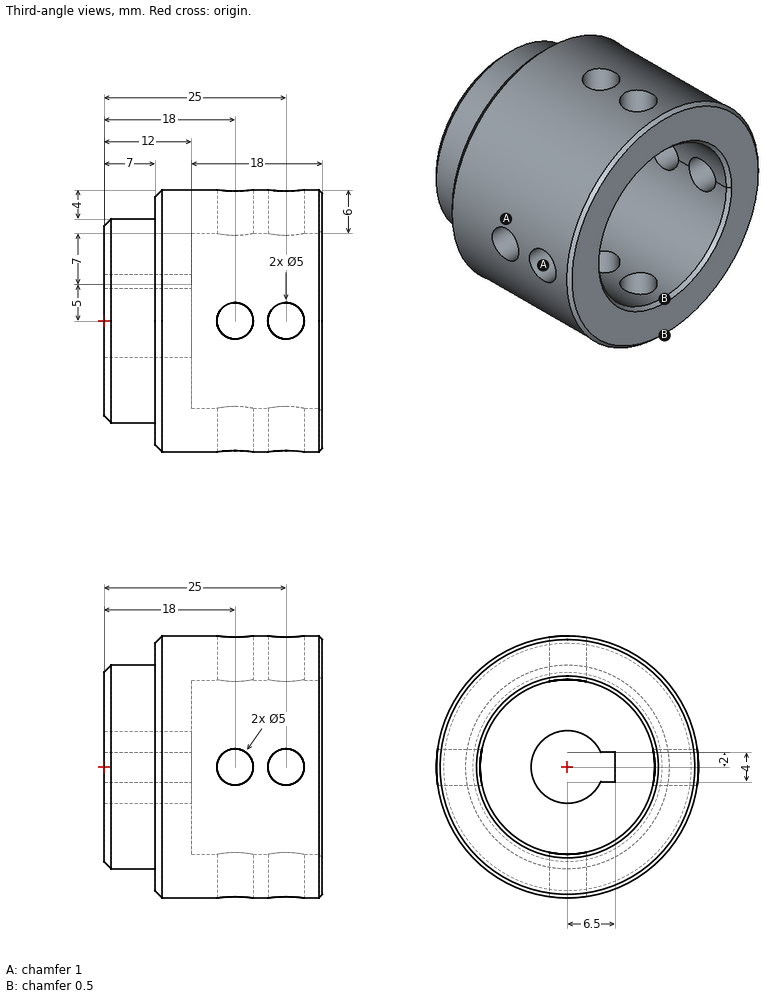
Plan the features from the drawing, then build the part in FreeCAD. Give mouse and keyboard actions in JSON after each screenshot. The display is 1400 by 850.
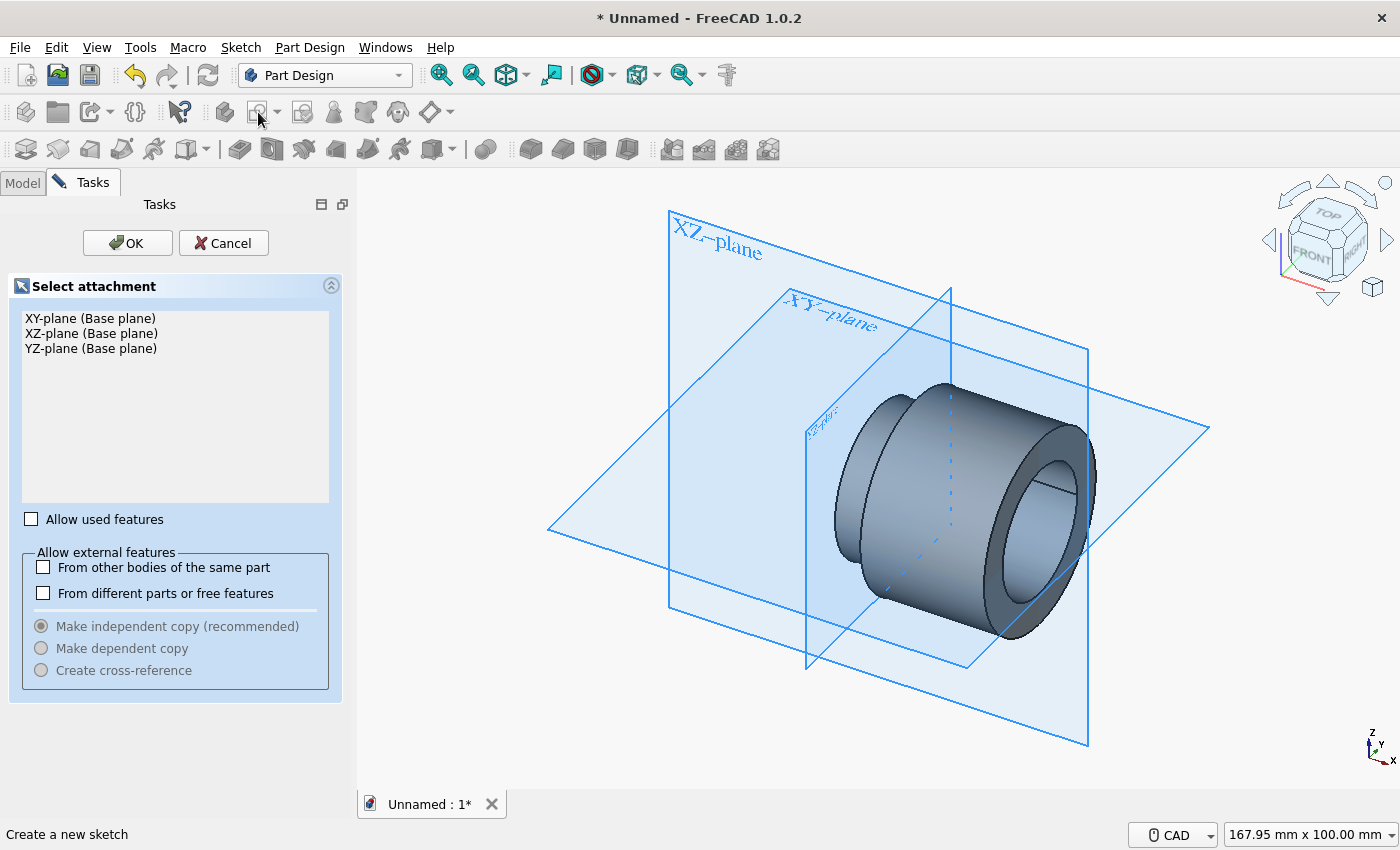
{"action": "left_click", "coordinate": [82, 334]}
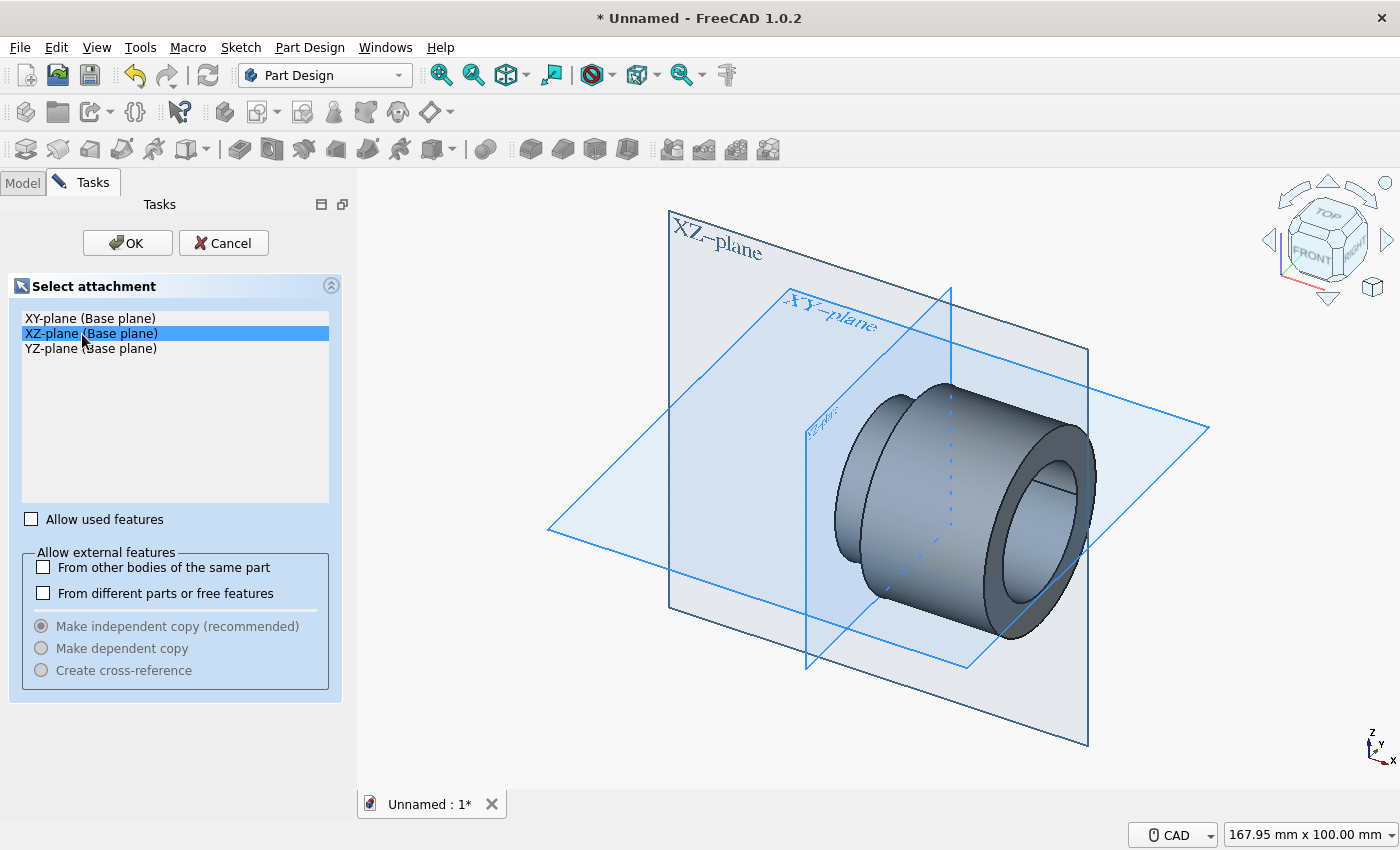
{"action": "left_click", "coordinate": [128, 243]}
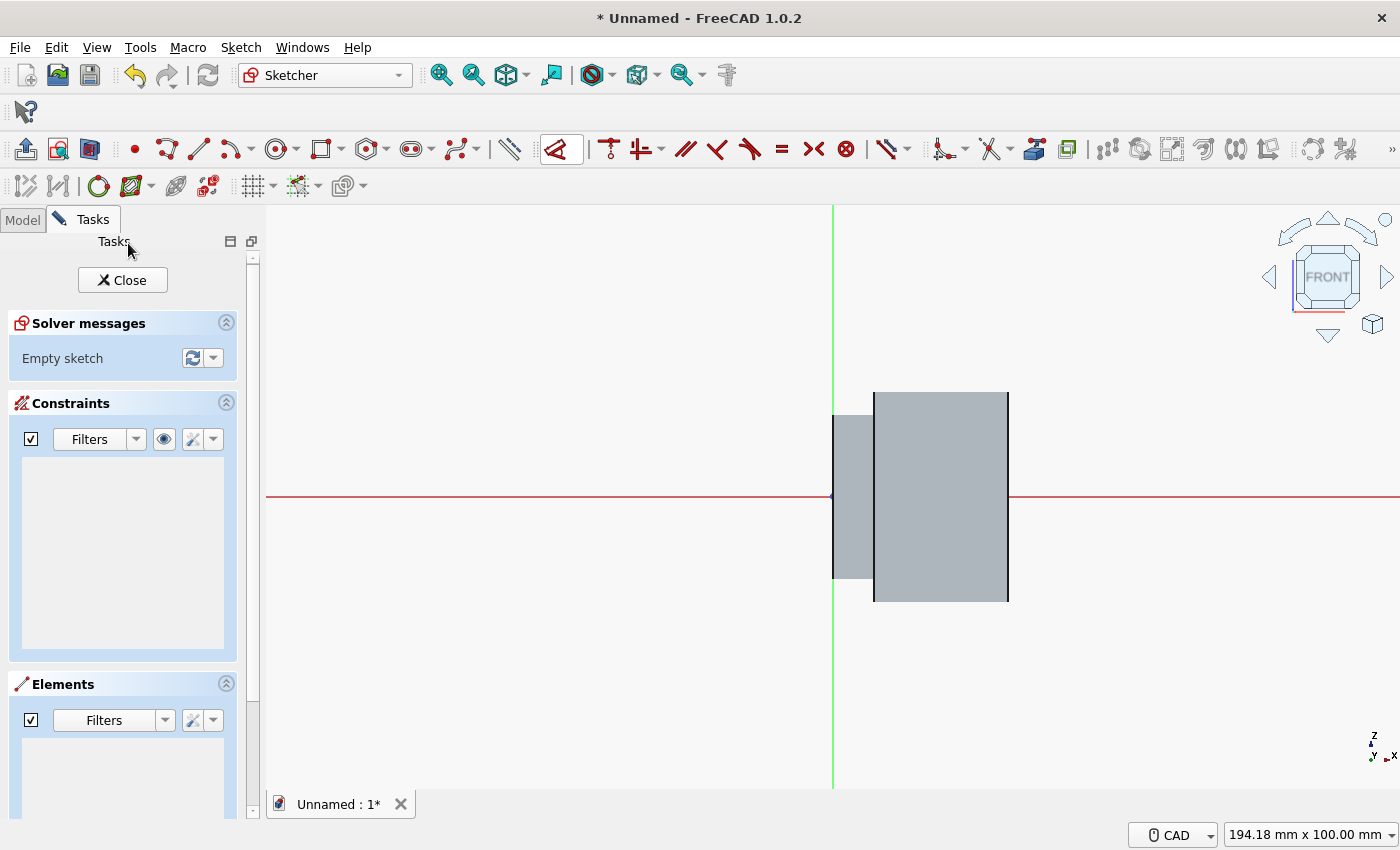
{"action": "left_click", "coordinate": [90, 150]}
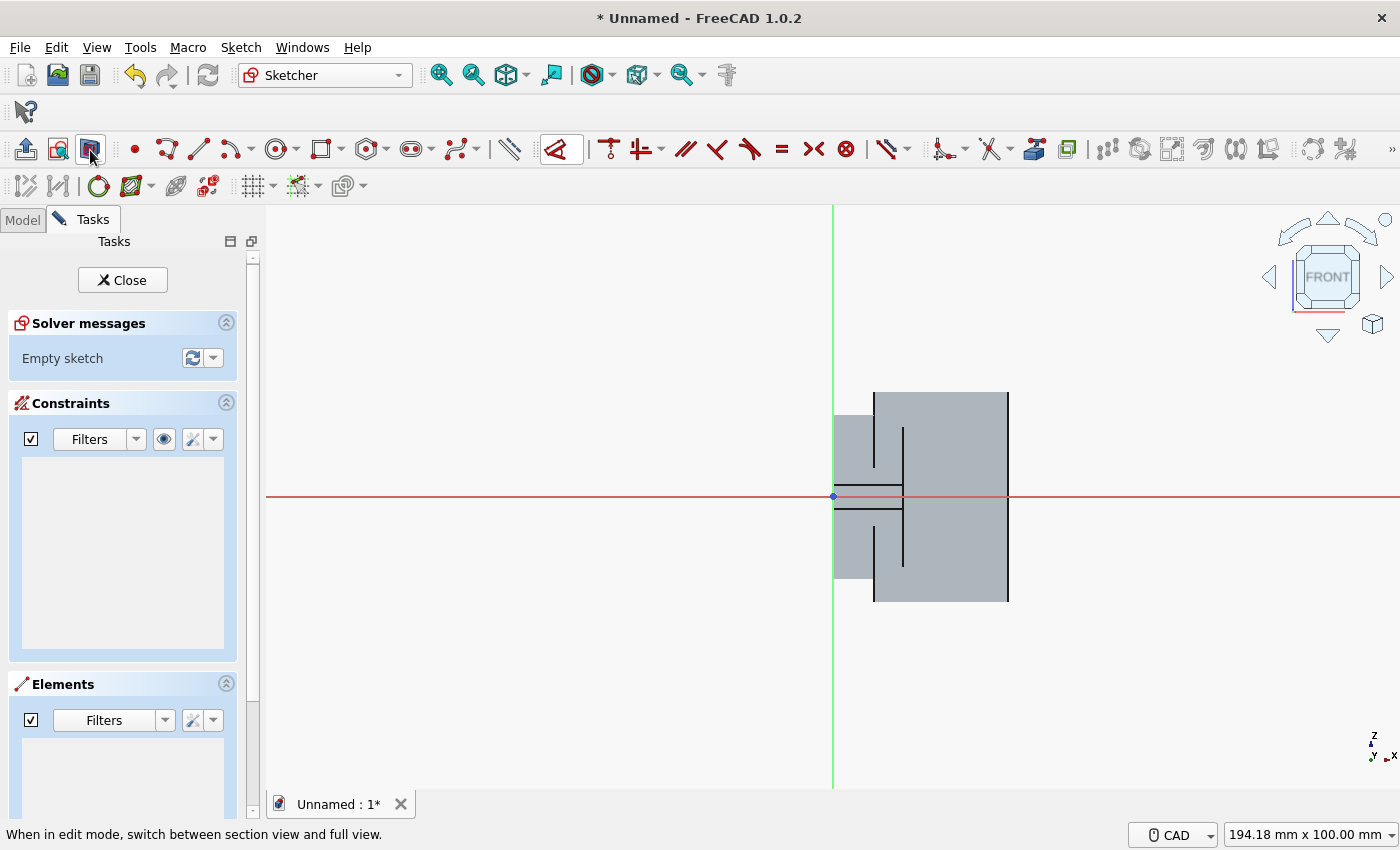
{"action": "scroll", "coordinate": [962, 497], "scroll_direction": "up", "scroll_amount": 7}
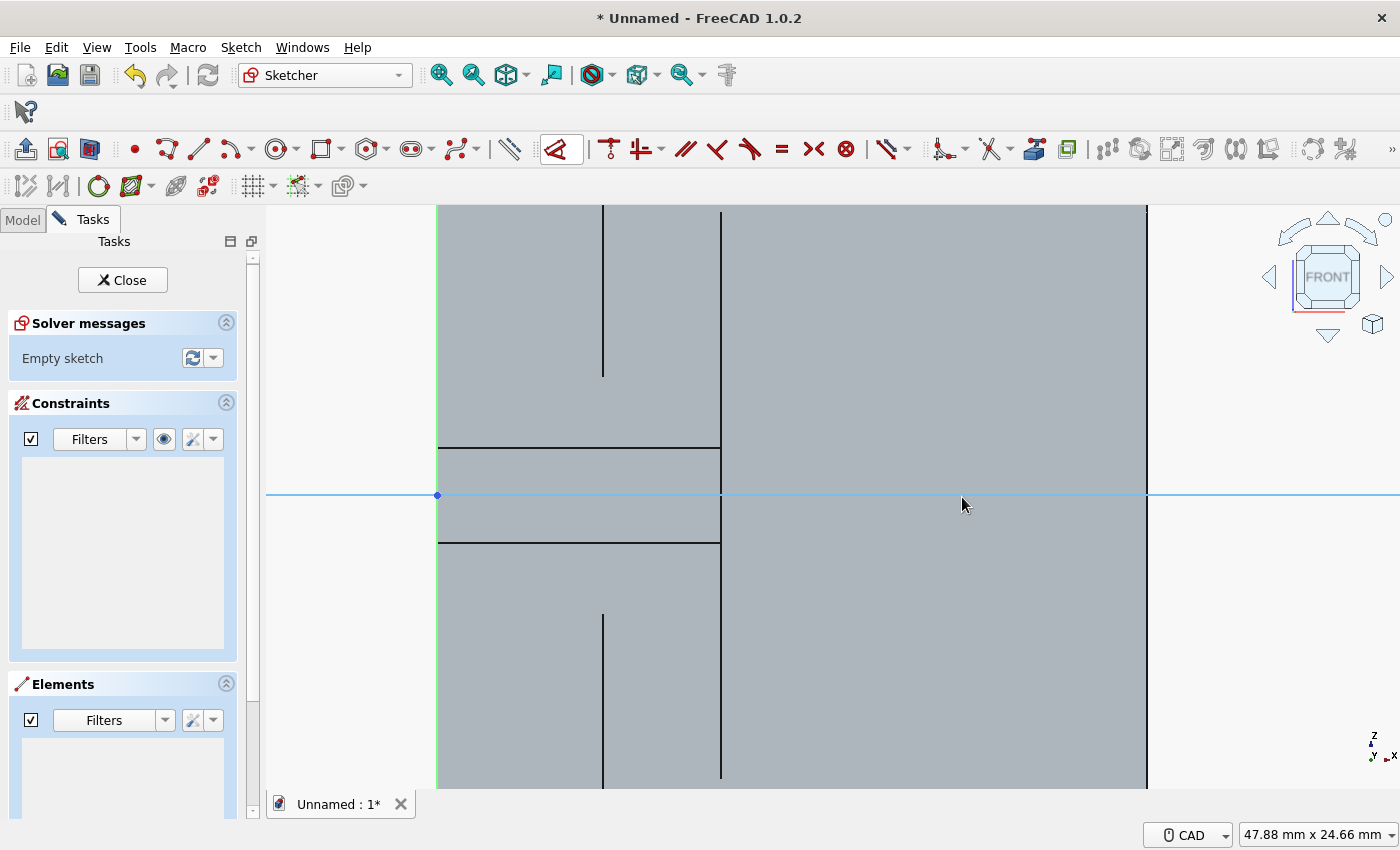
{"action": "left_click", "coordinate": [276, 150]}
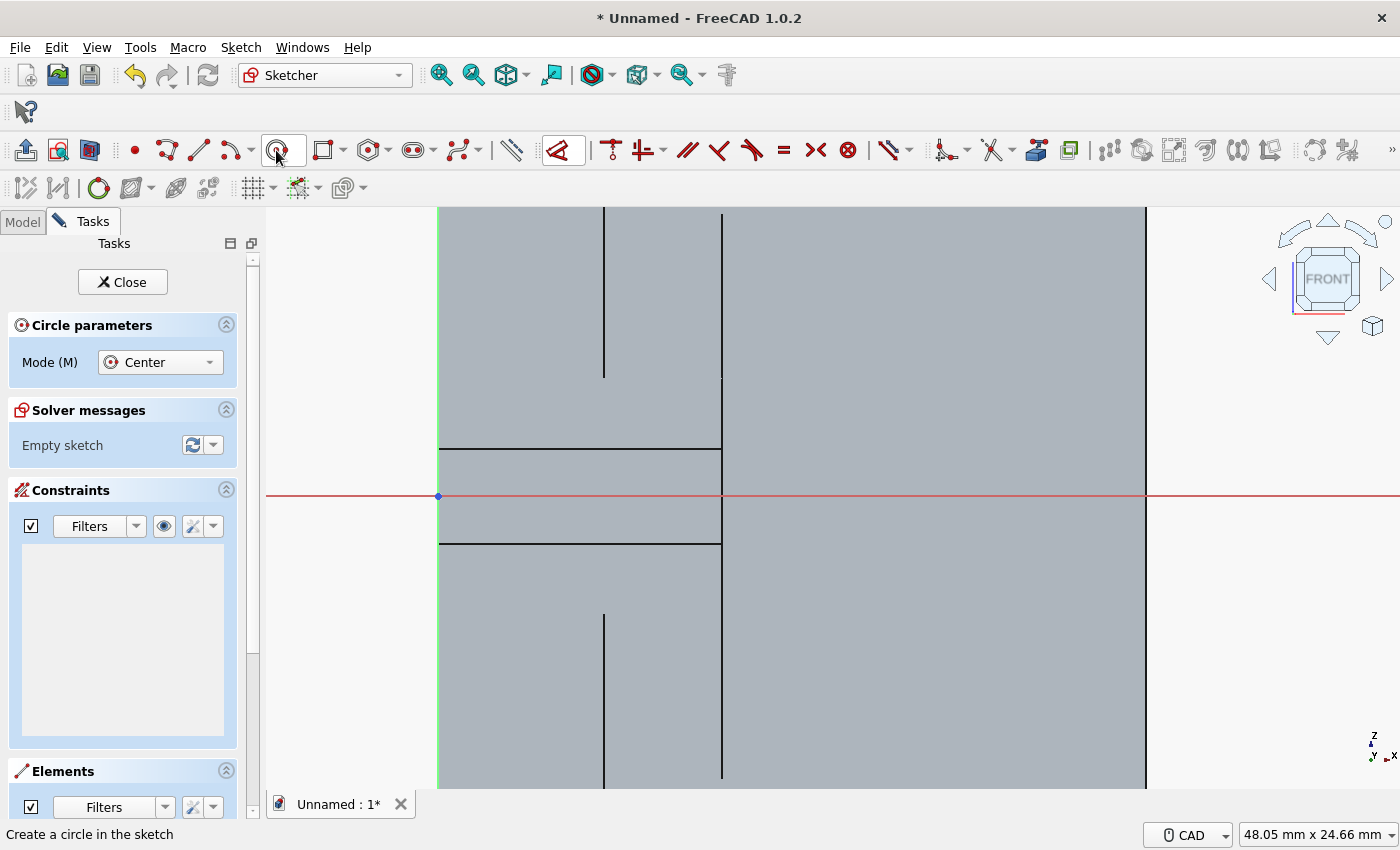
{"action": "left_click", "coordinate": [863, 496]}
{"action": "left_click", "coordinate": [905, 455]}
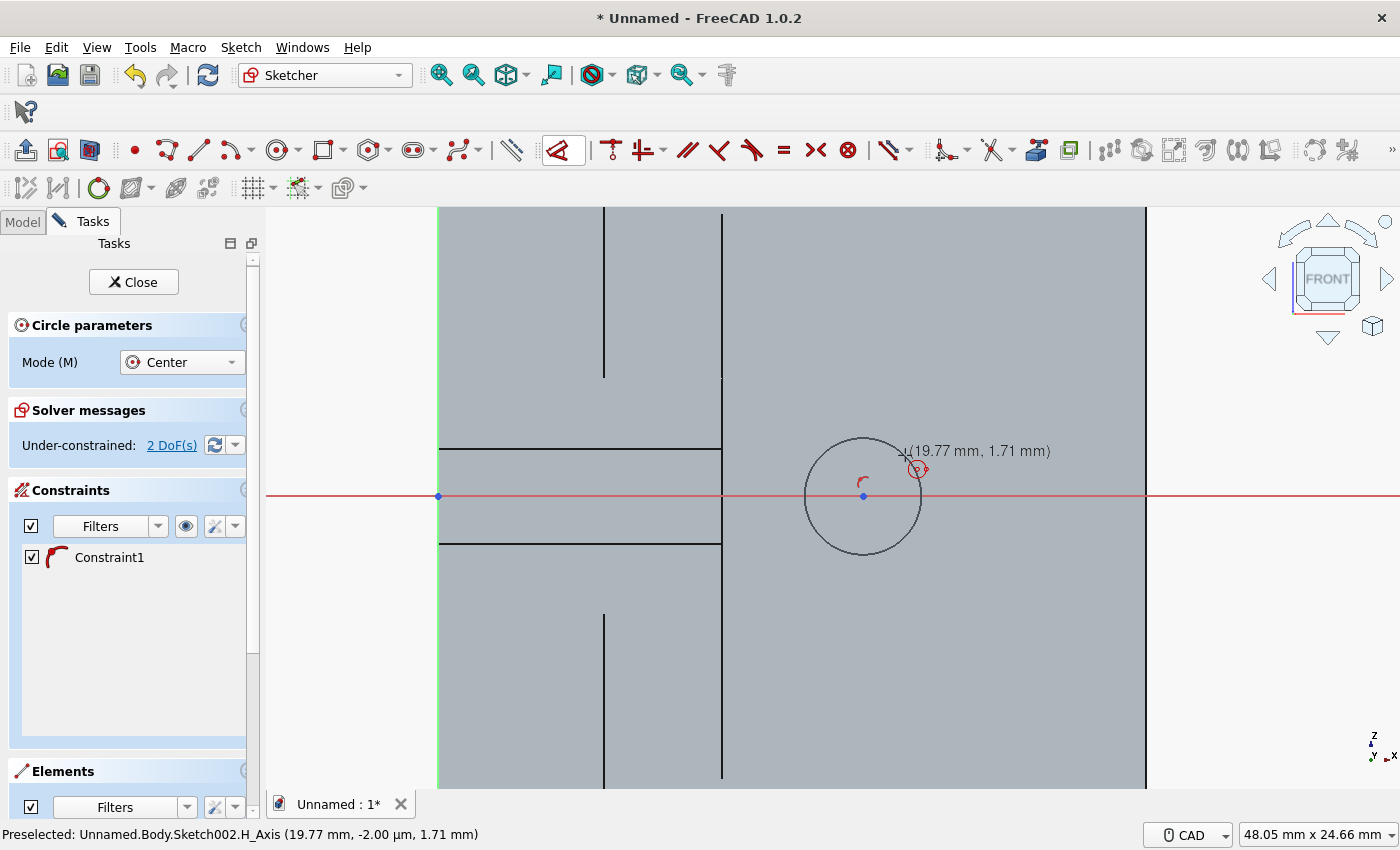
{"action": "left_click", "coordinate": [1028, 496]}
{"action": "left_click", "coordinate": [1070, 455]}
{"action": "key", "text": "Escape"}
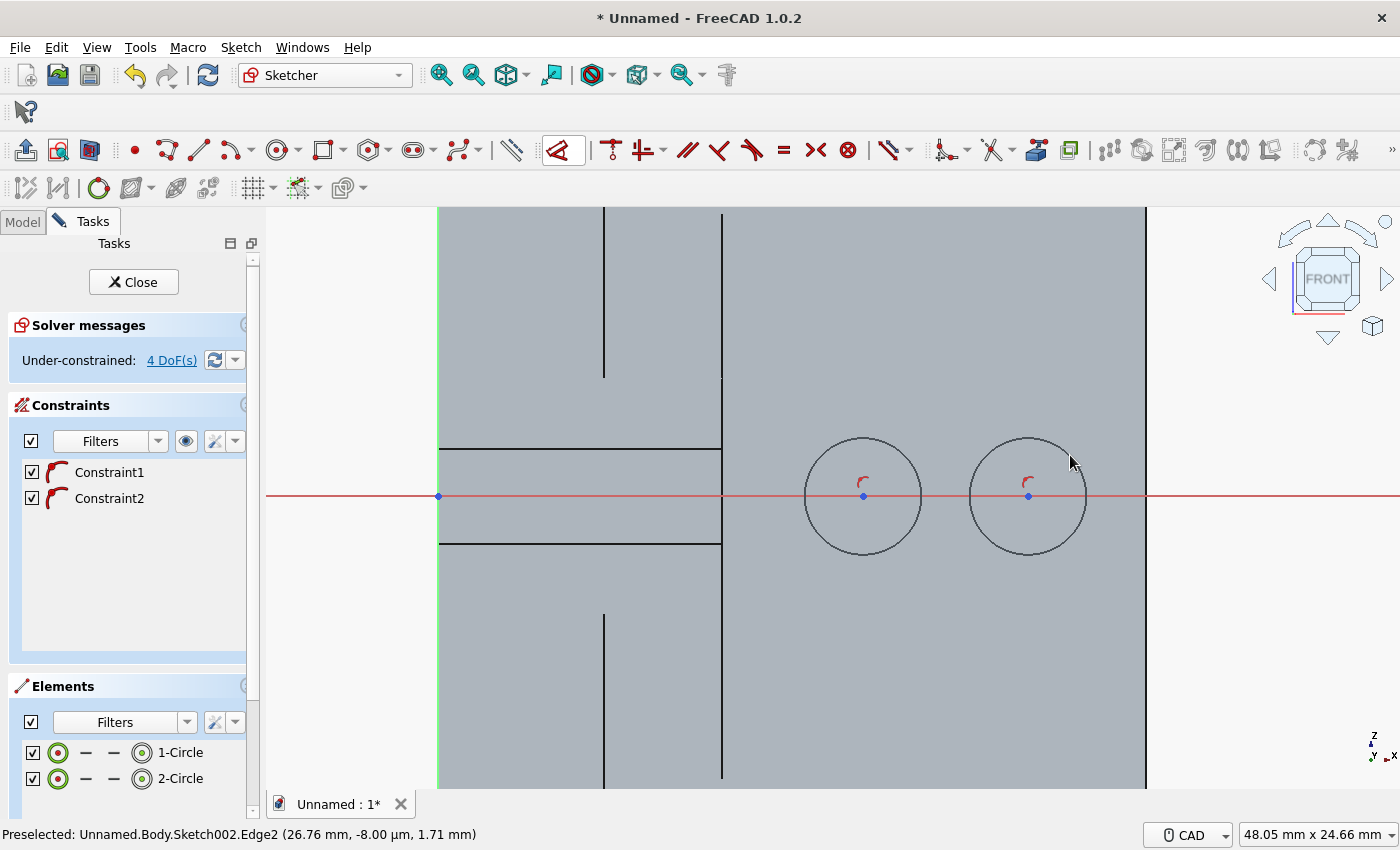
{"action": "left_click", "coordinate": [904, 455]}